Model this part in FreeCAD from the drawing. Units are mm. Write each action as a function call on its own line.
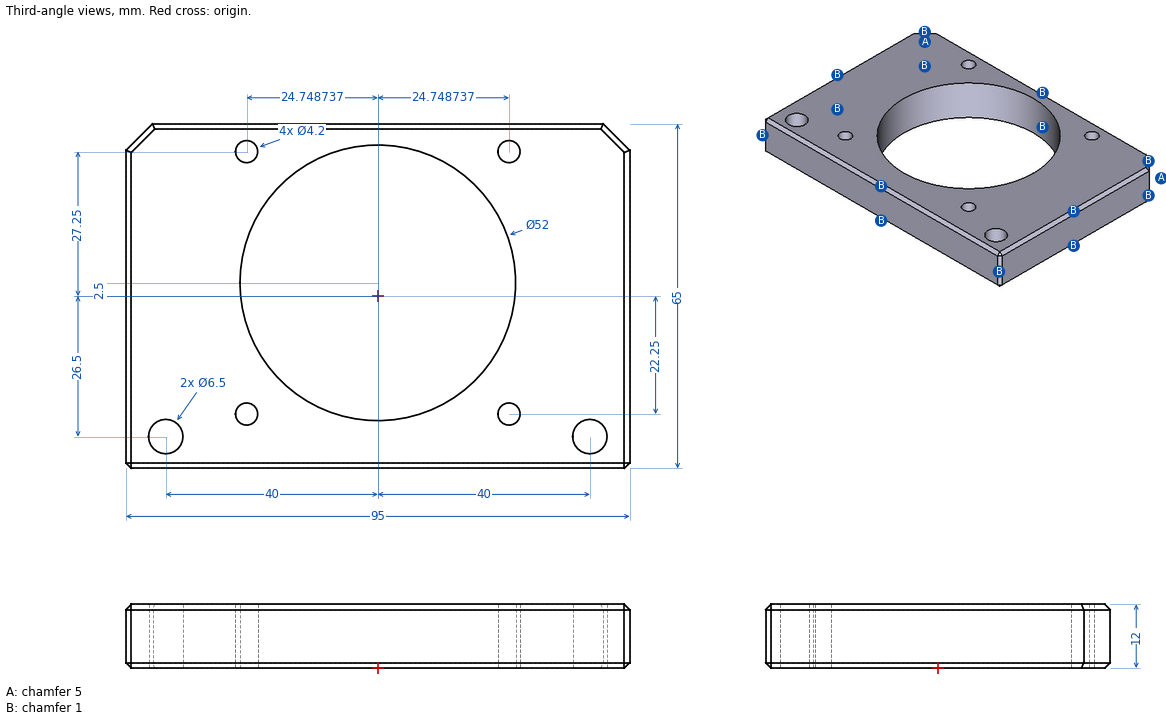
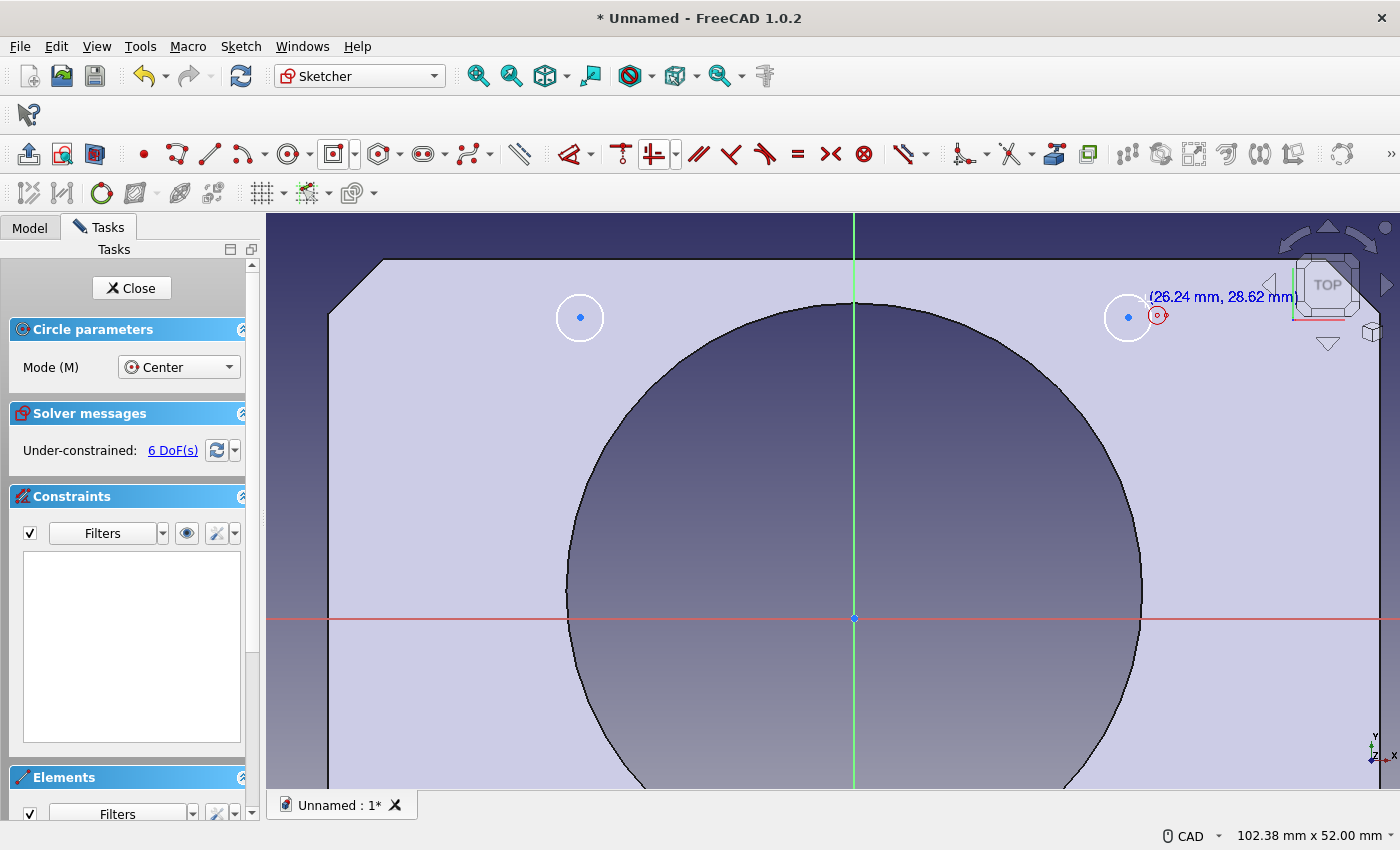
scroll(582, 317, down, 2)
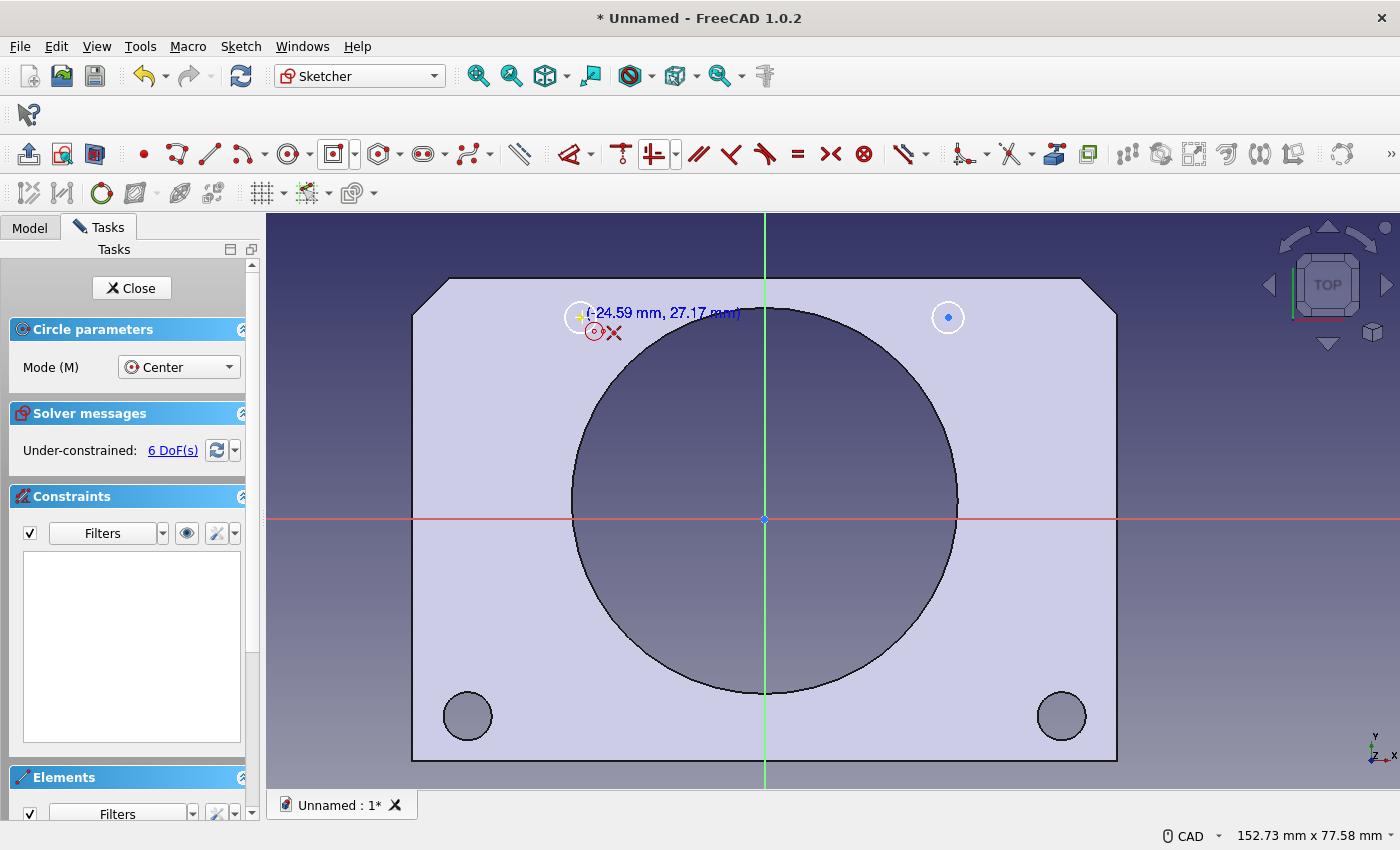
scroll(948, 685, up, 2)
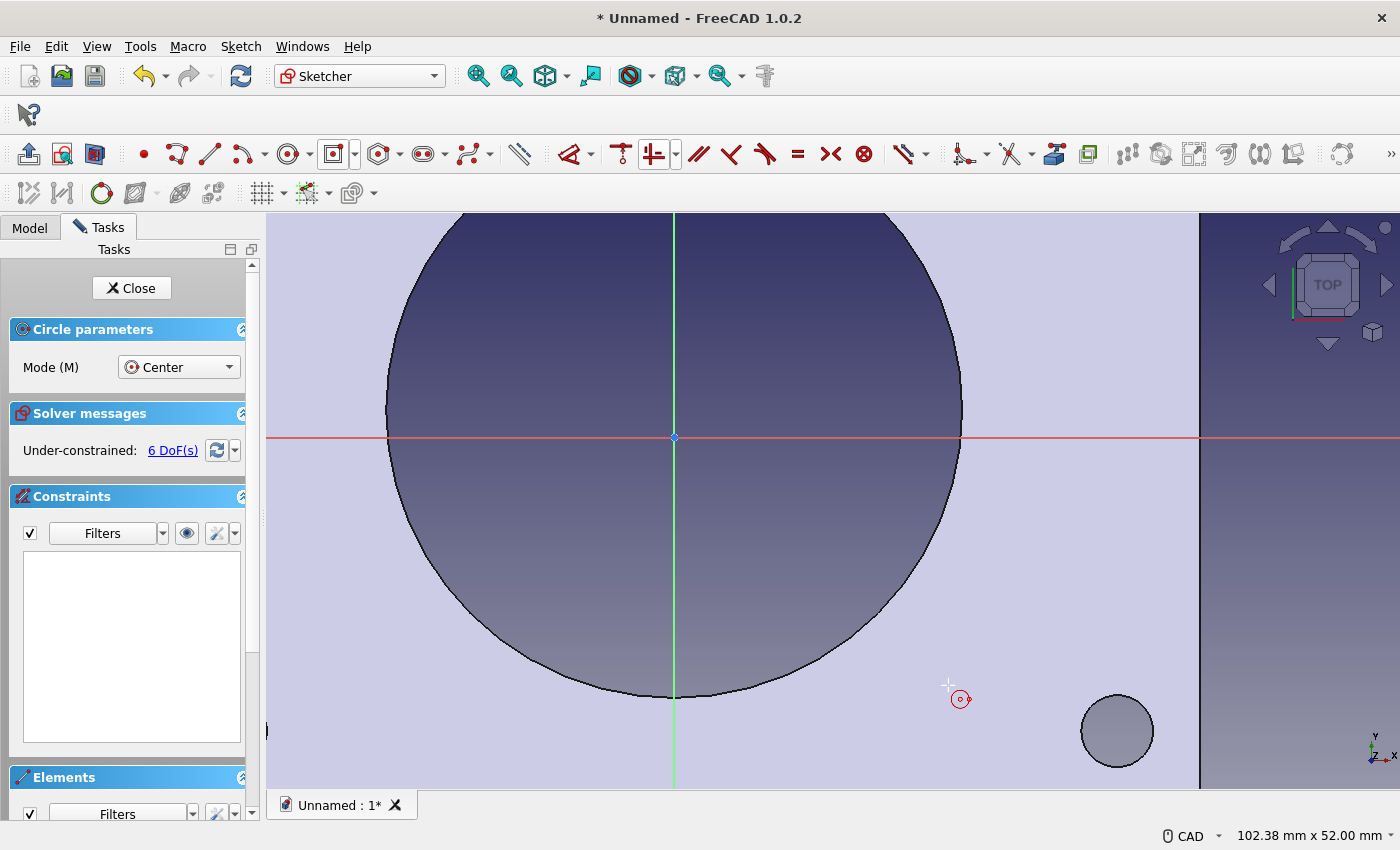
click(948, 684)
click(965, 668)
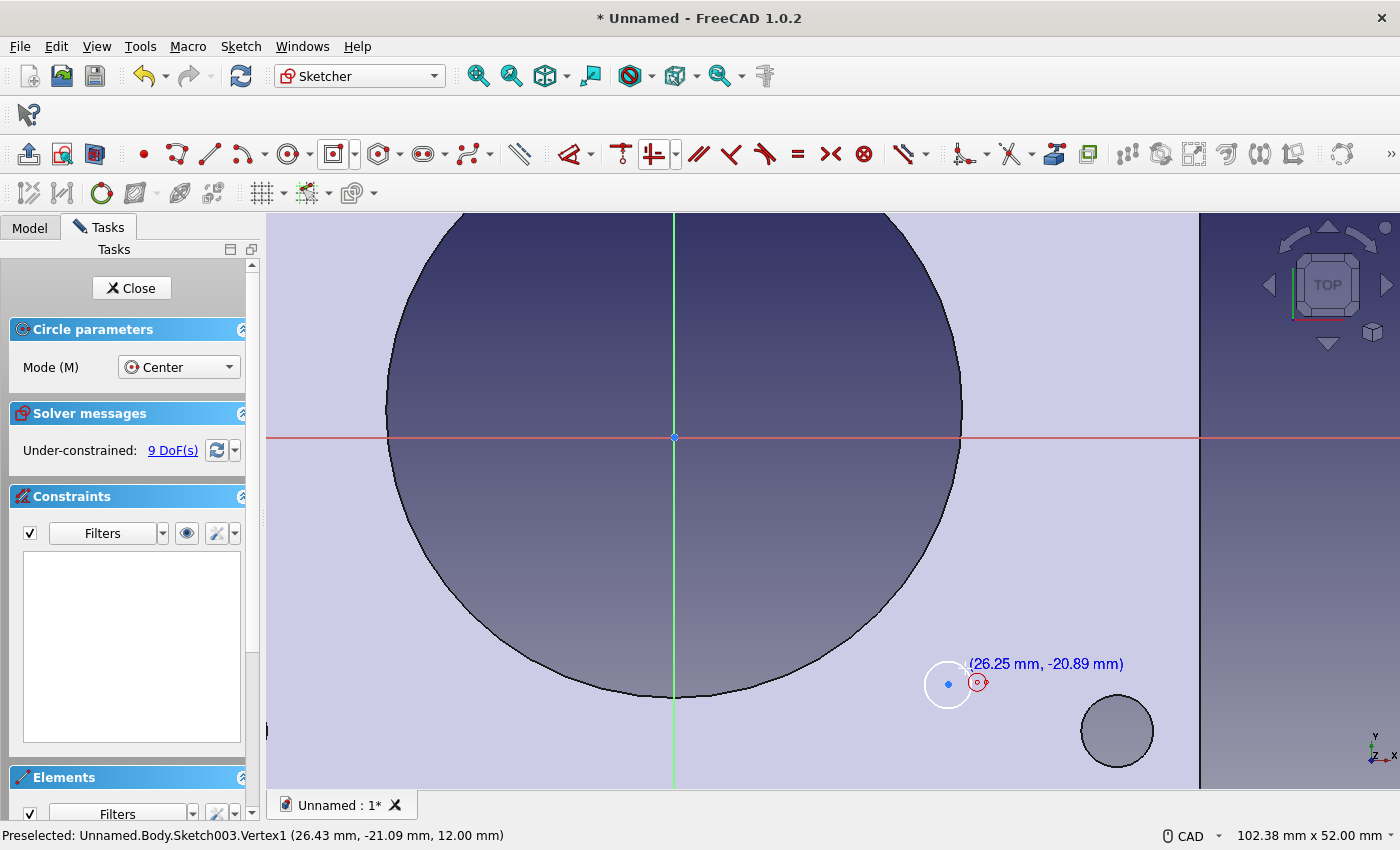
click(400, 684)
click(417, 668)
key(Escape)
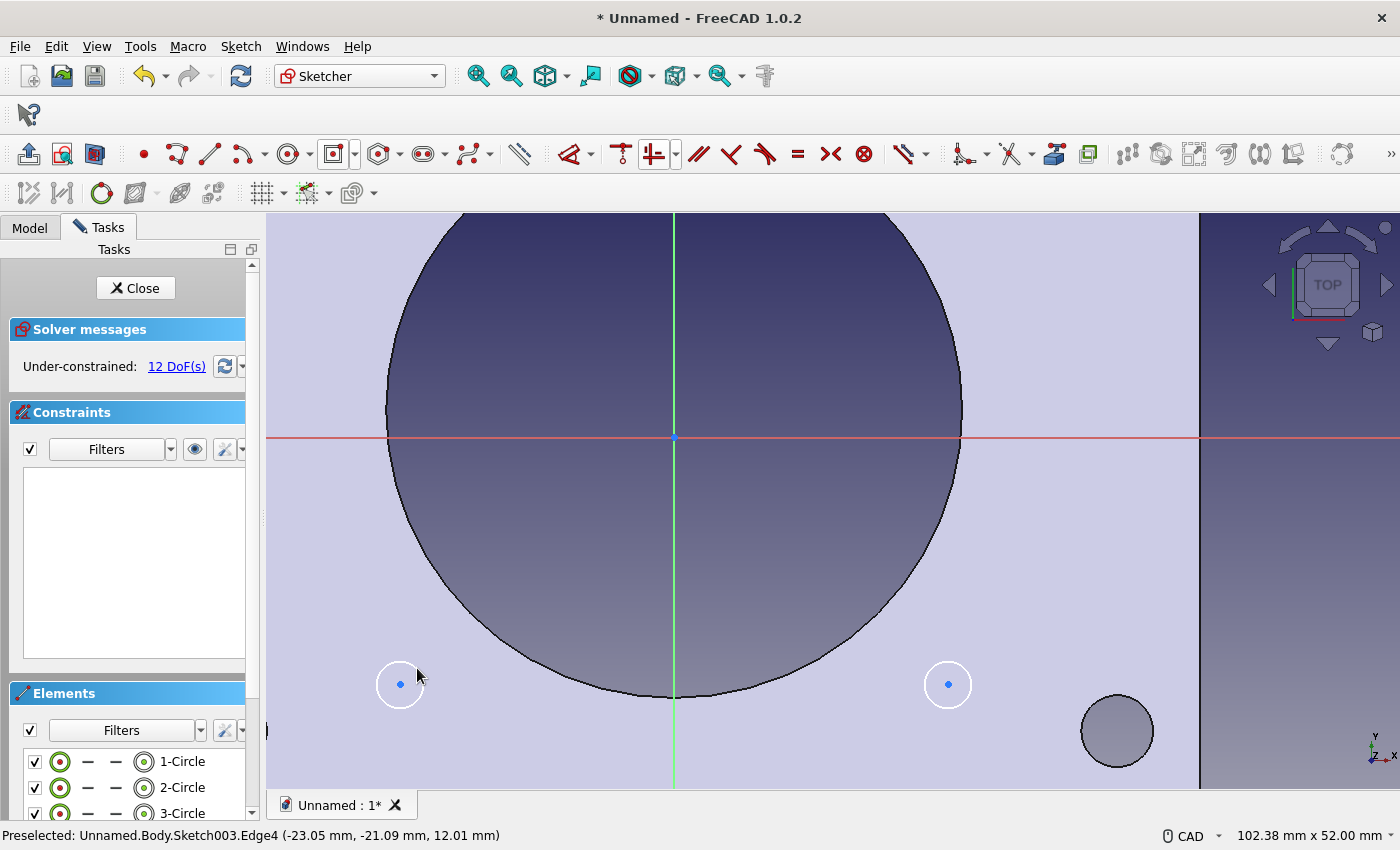
scroll(948, 686, down, 2)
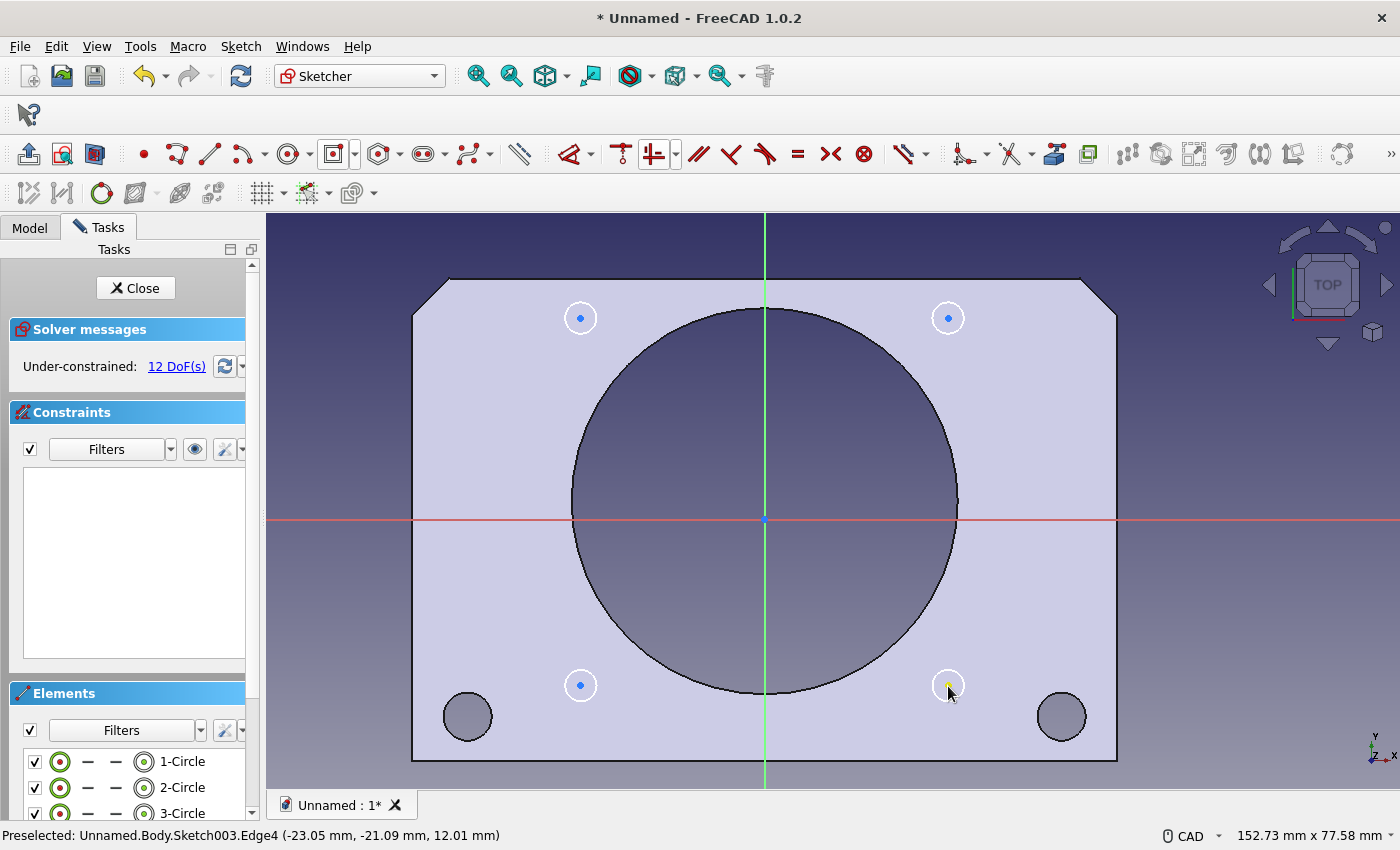
click(592, 307)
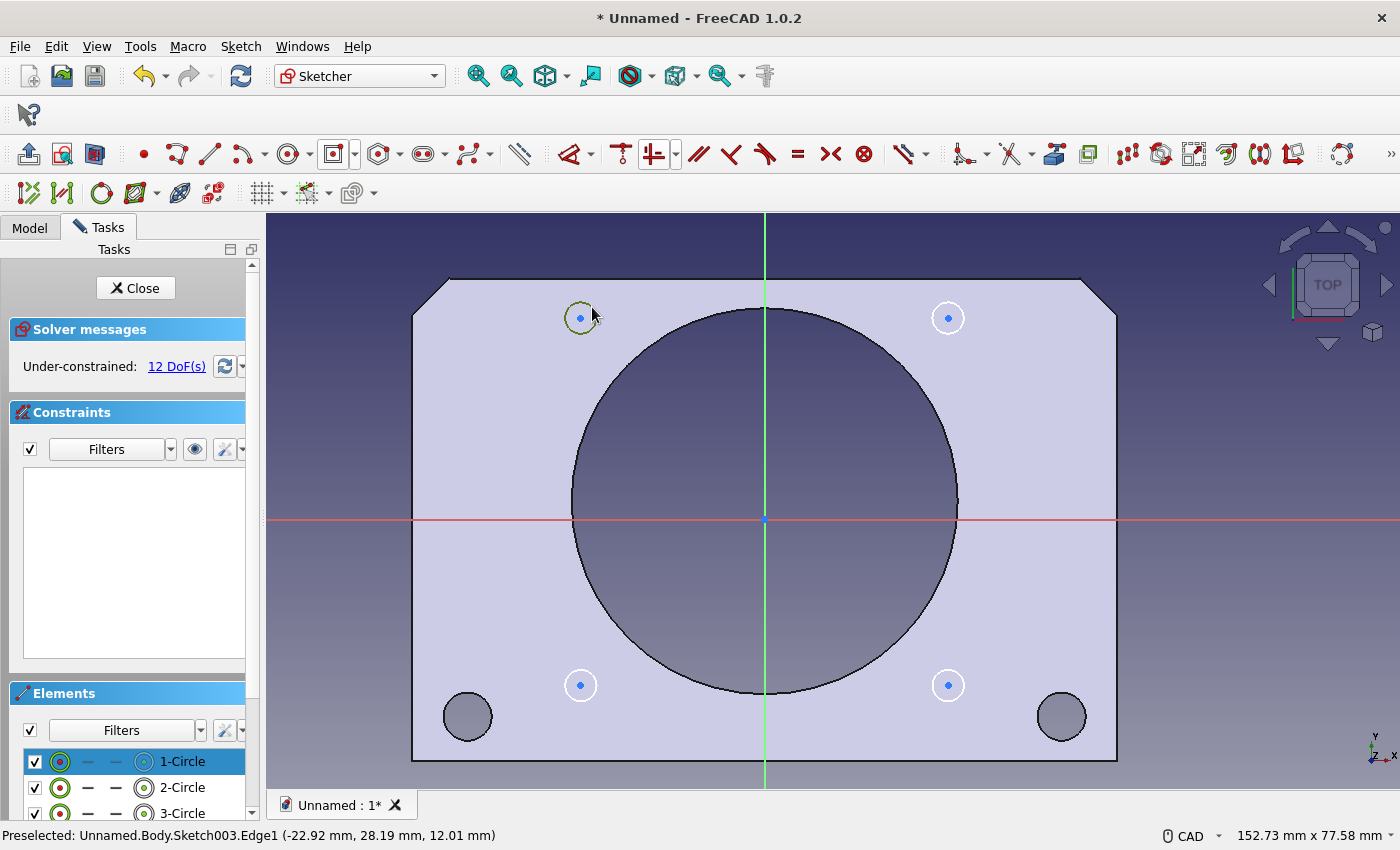
click(959, 307)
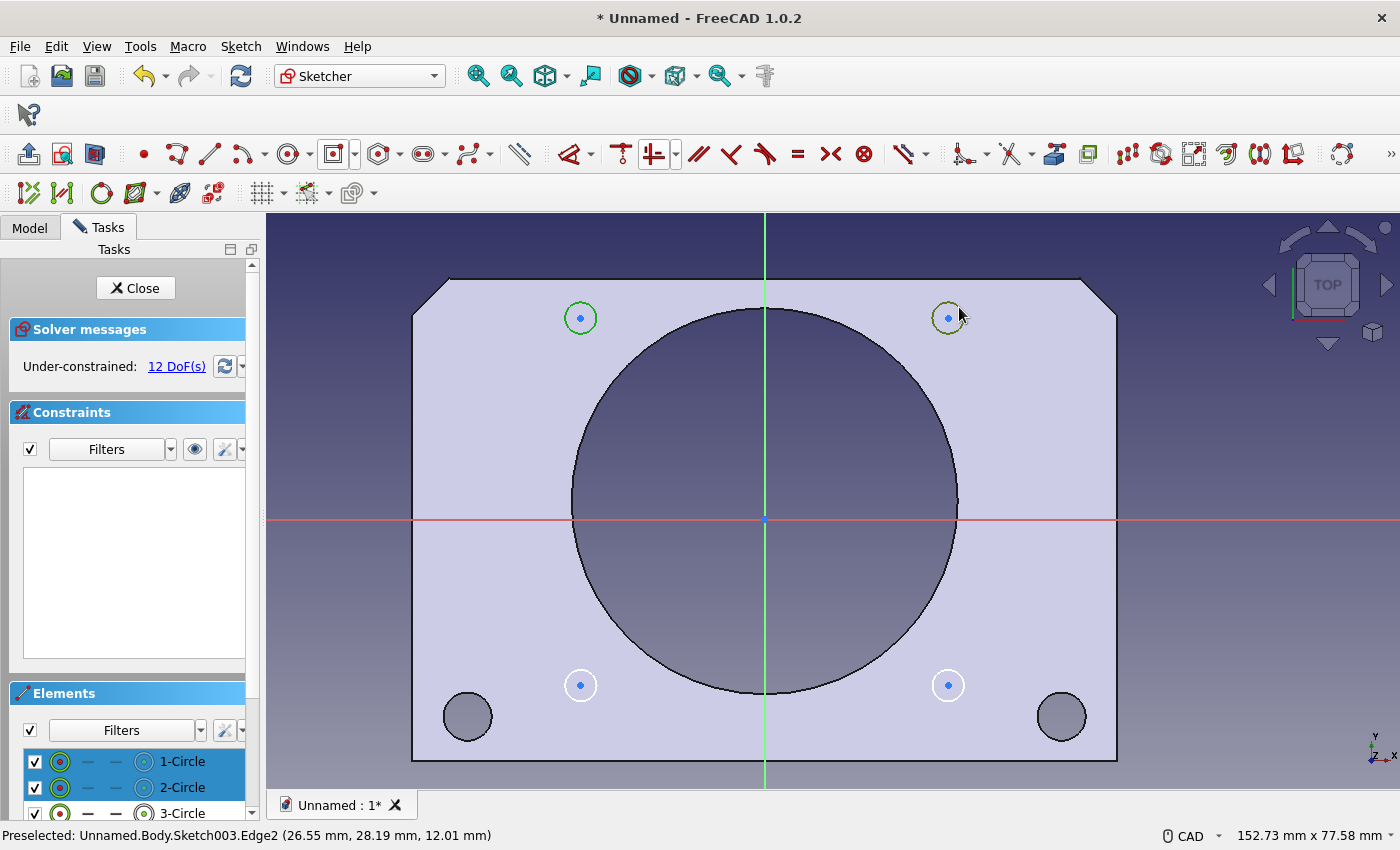
click(959, 675)